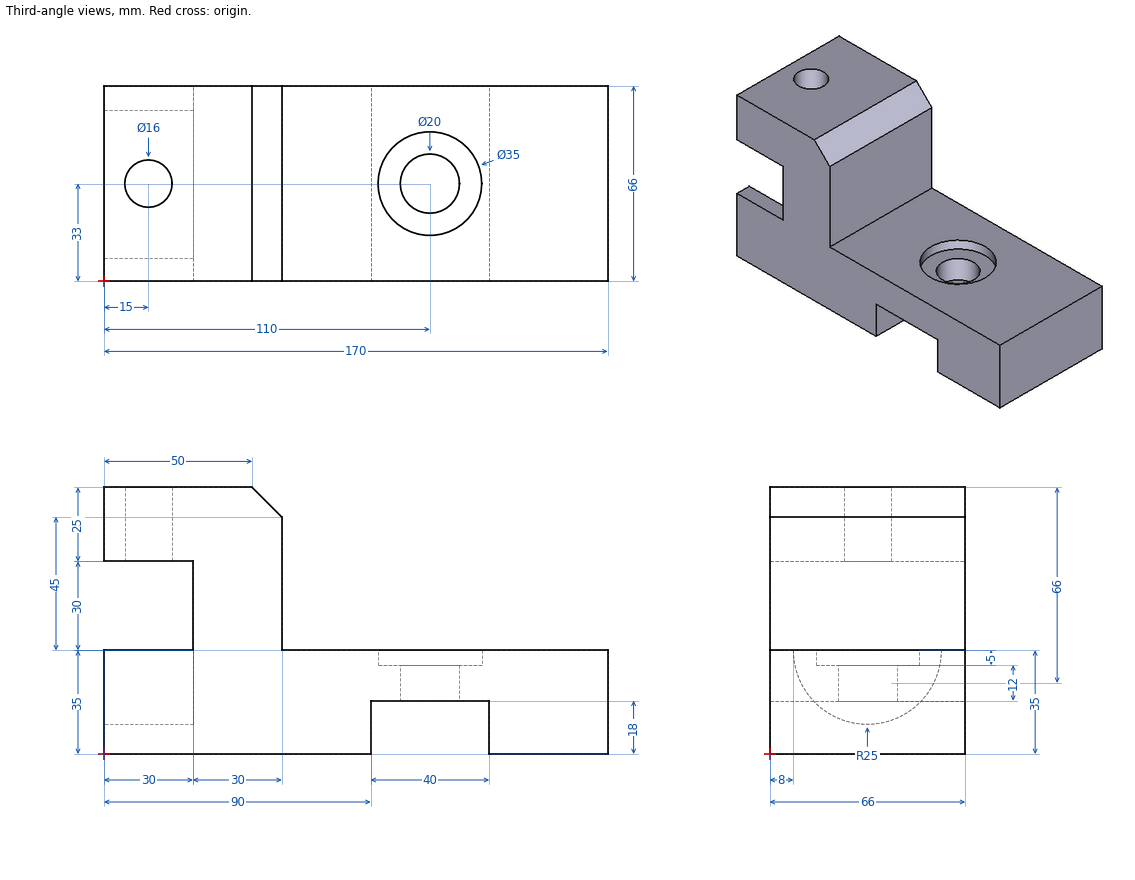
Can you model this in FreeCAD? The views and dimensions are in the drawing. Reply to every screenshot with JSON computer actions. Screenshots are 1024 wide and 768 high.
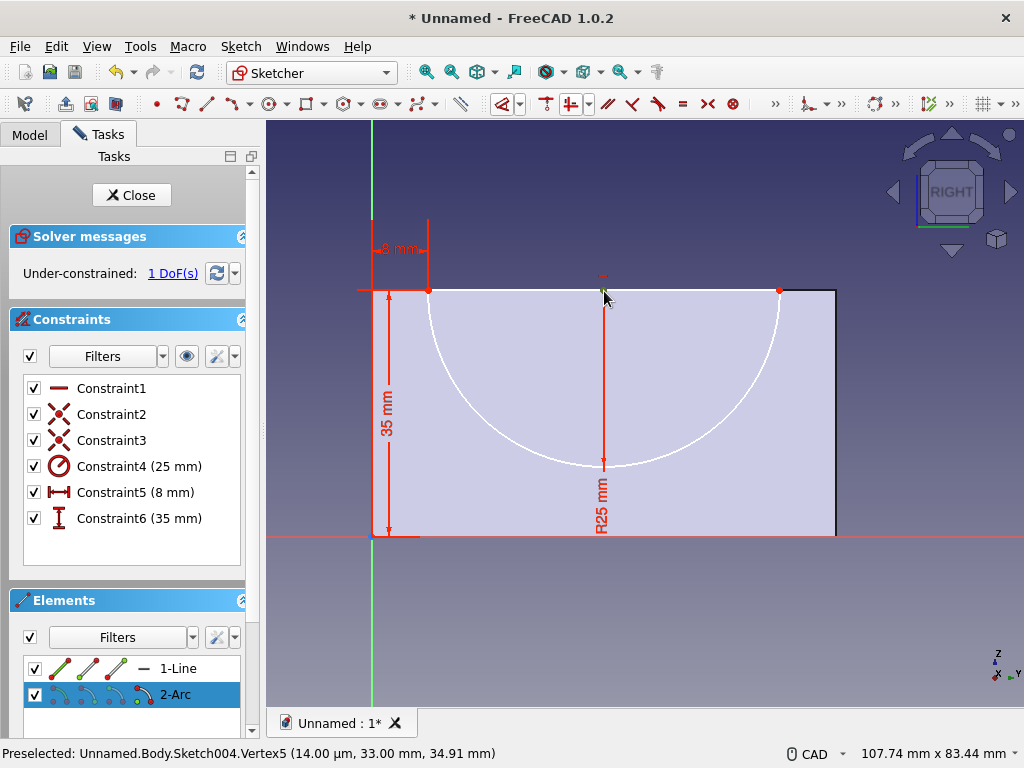
{"action": "left_click", "coordinate": [520, 104]}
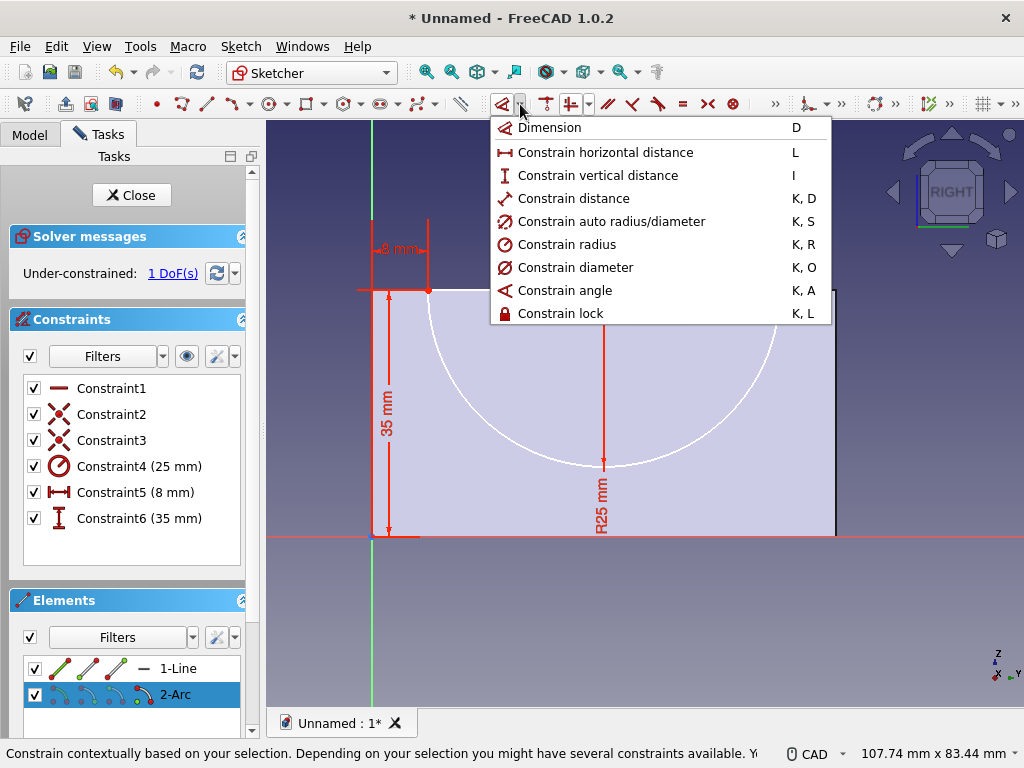
{"action": "left_click", "coordinate": [661, 176]}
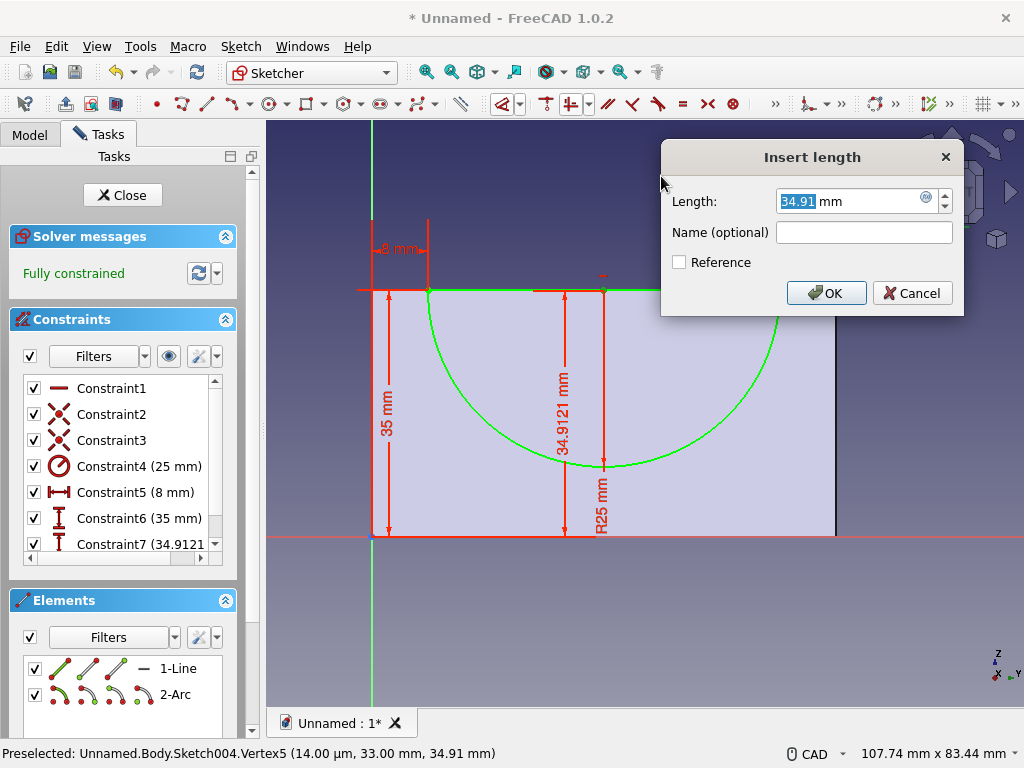
{"action": "type", "text": "35"}
{"action": "key", "text": "Return"}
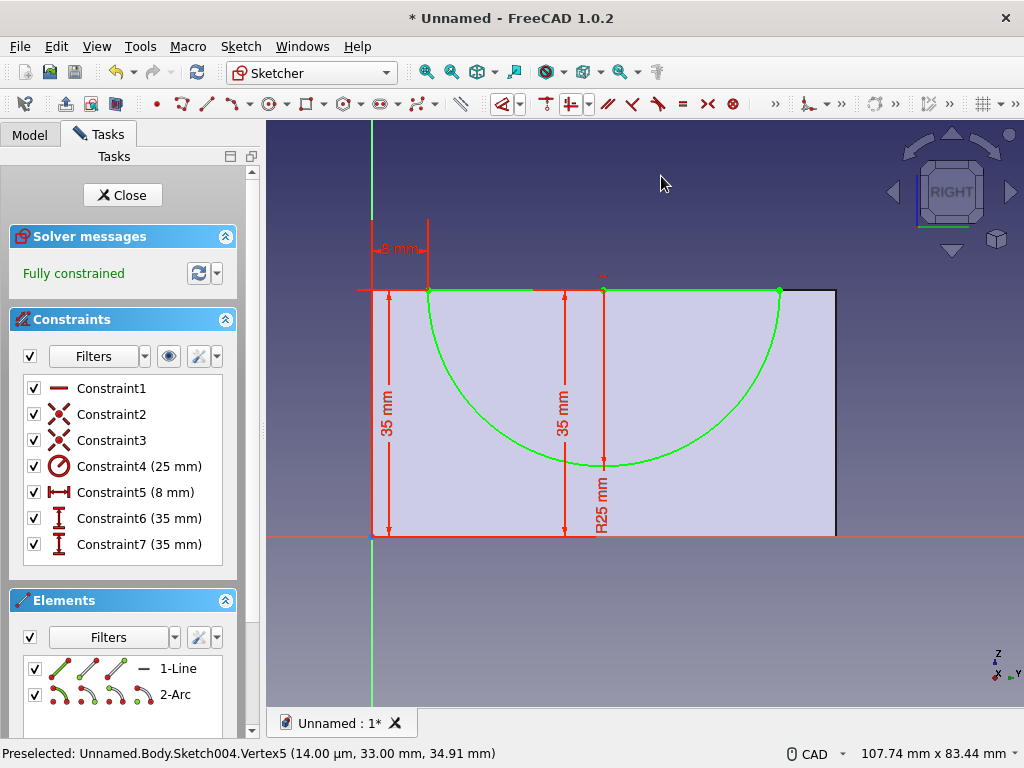
{"action": "left_click", "coordinate": [123, 195]}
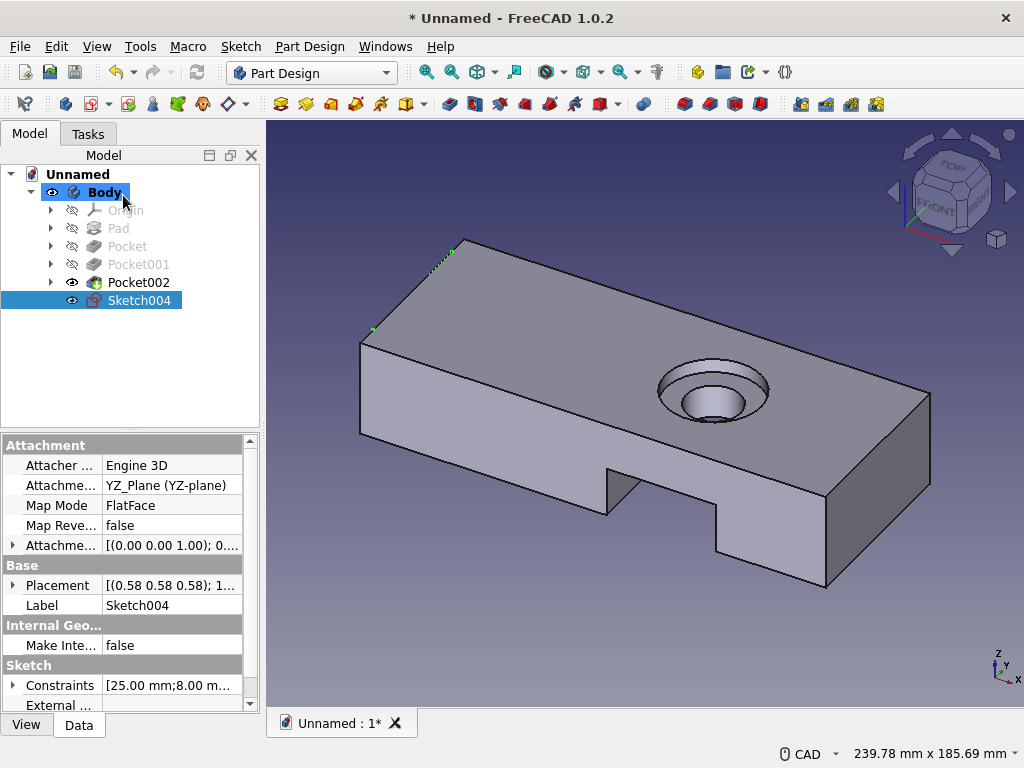
{"action": "left_click", "coordinate": [450, 104]}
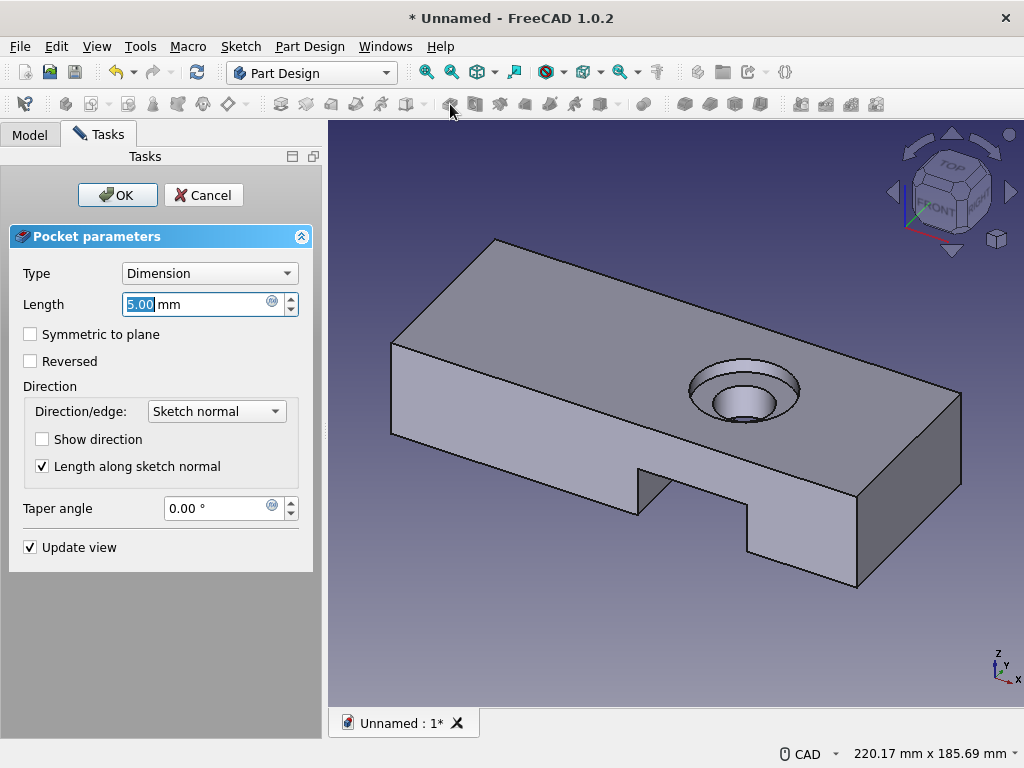
{"action": "type", "text": "30"}
{"action": "key", "text": "Tab"}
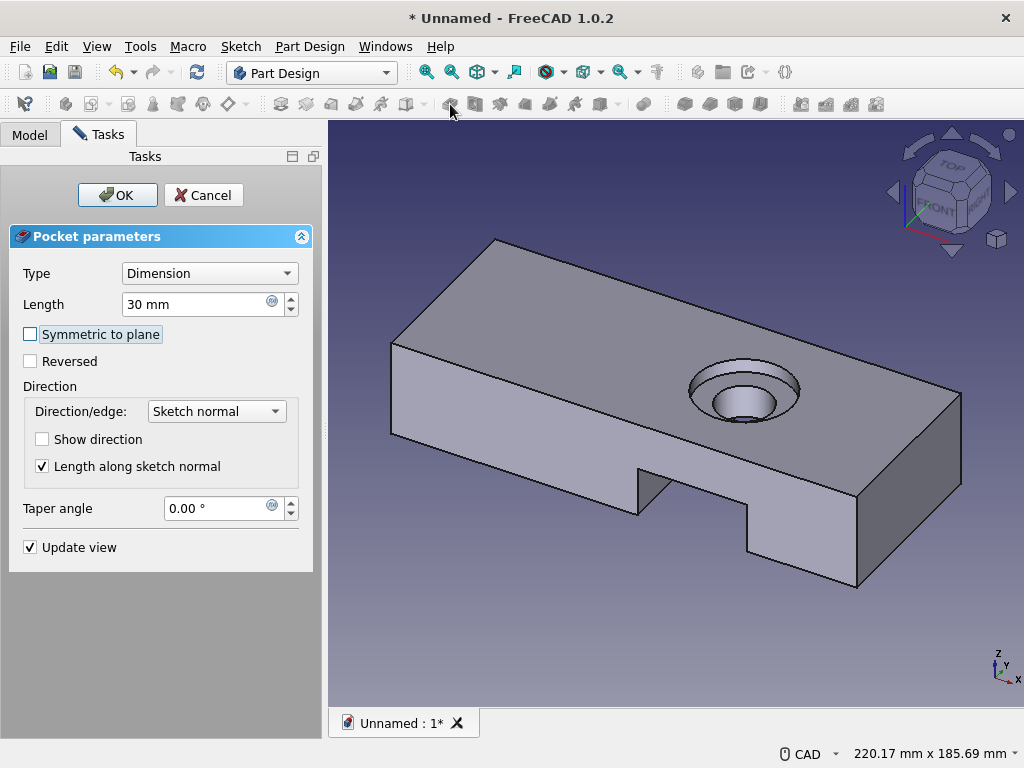
{"action": "left_click", "coordinate": [31, 361]}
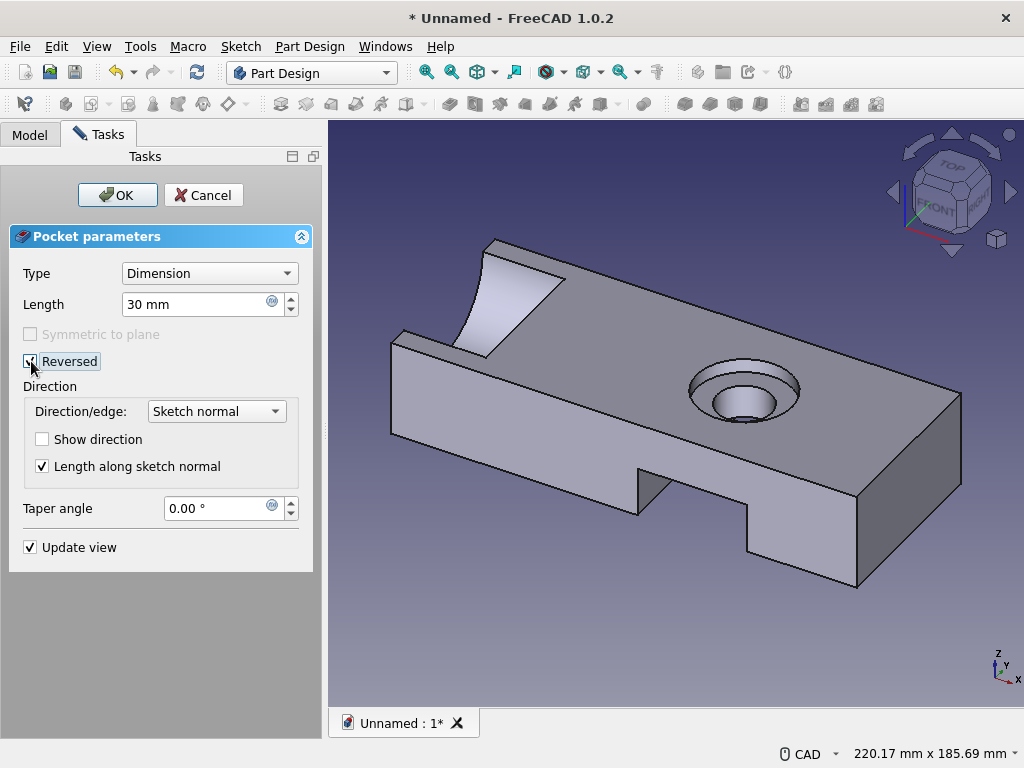
{"action": "left_click", "coordinate": [118, 195]}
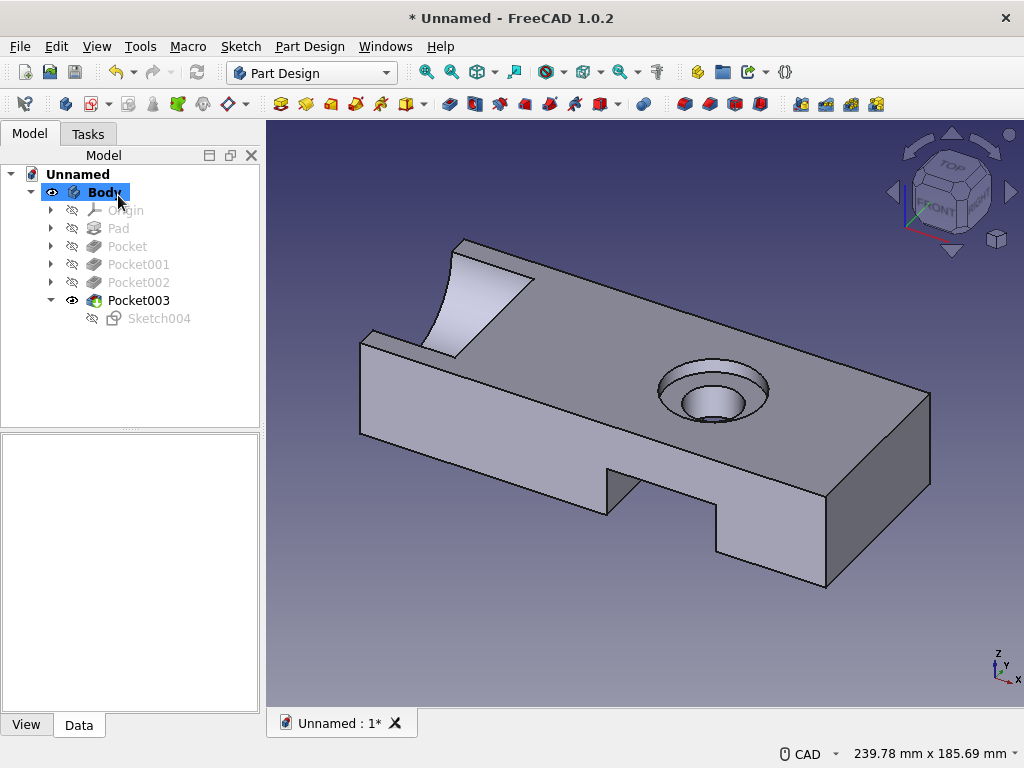
{"action": "left_click", "coordinate": [90, 104]}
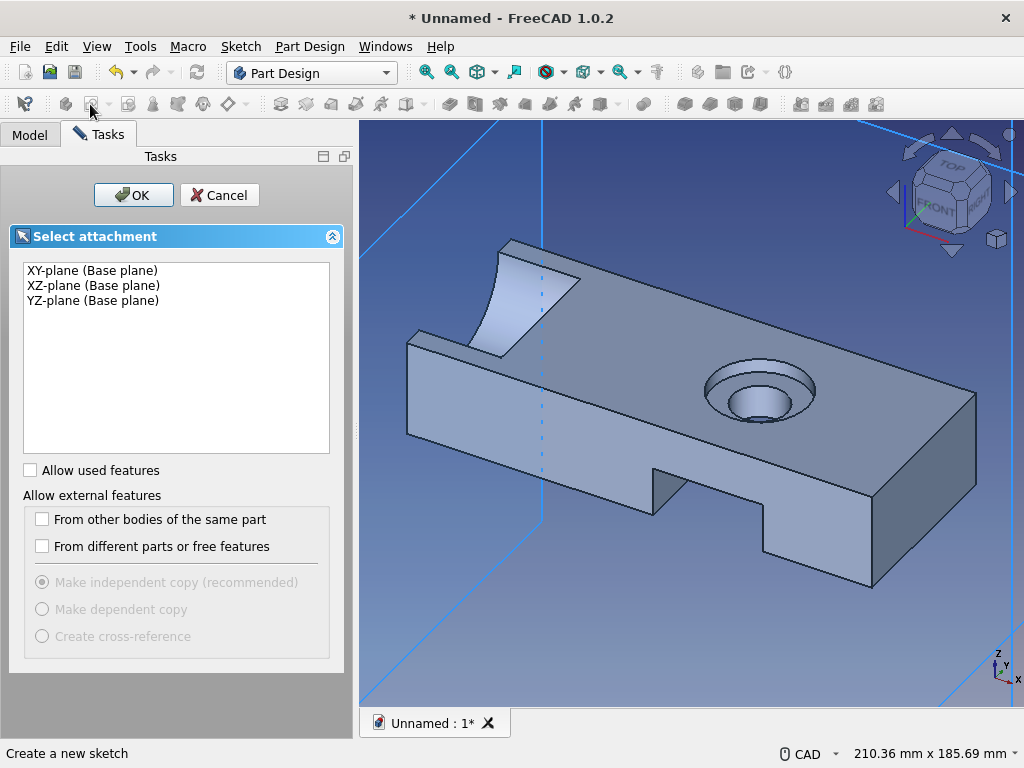
{"action": "left_click", "coordinate": [84, 286]}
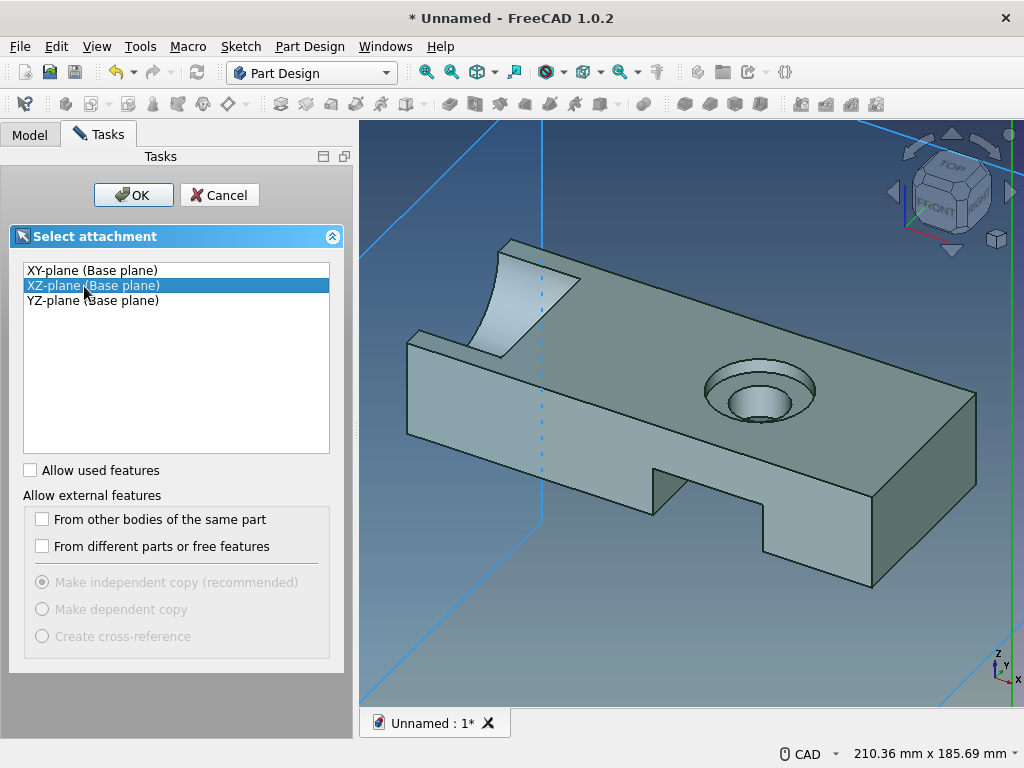
{"action": "left_click", "coordinate": [134, 195]}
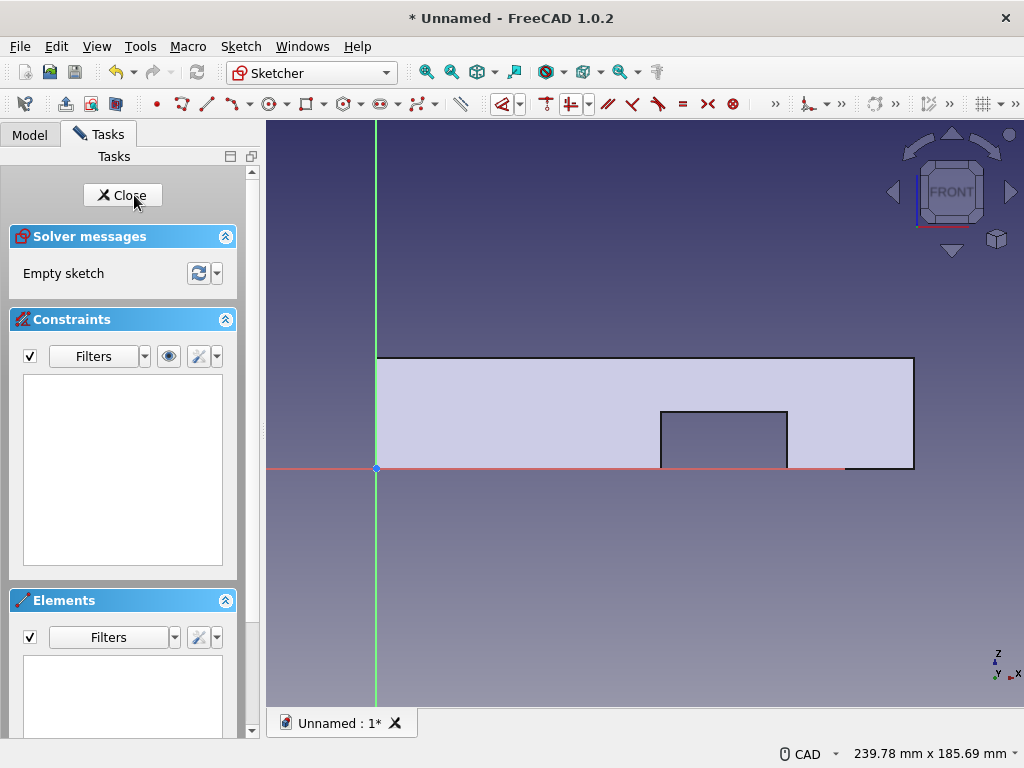
{"action": "key", "text": "g m"}